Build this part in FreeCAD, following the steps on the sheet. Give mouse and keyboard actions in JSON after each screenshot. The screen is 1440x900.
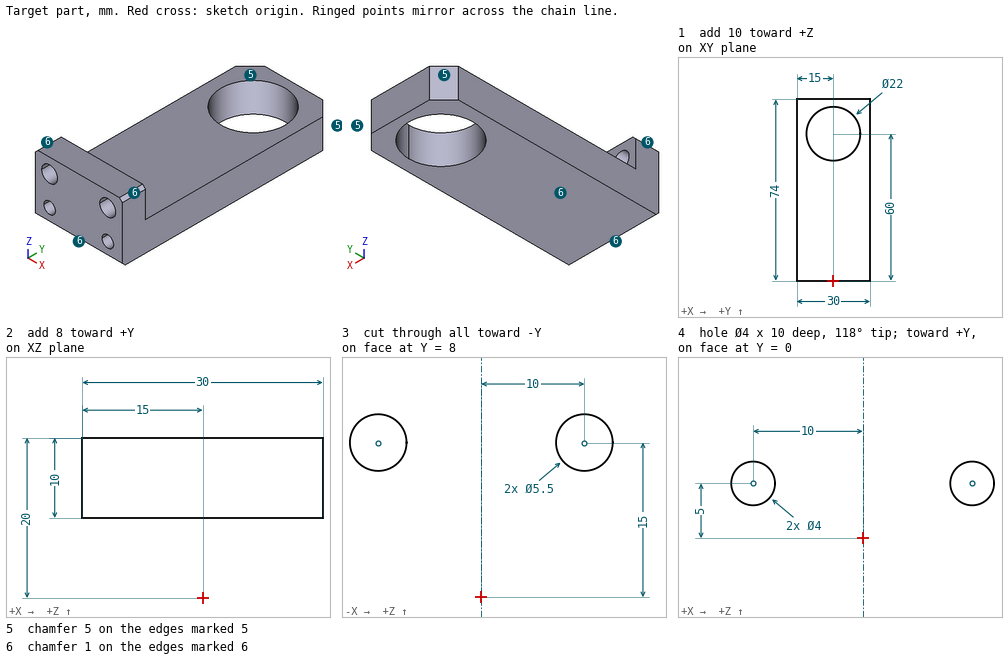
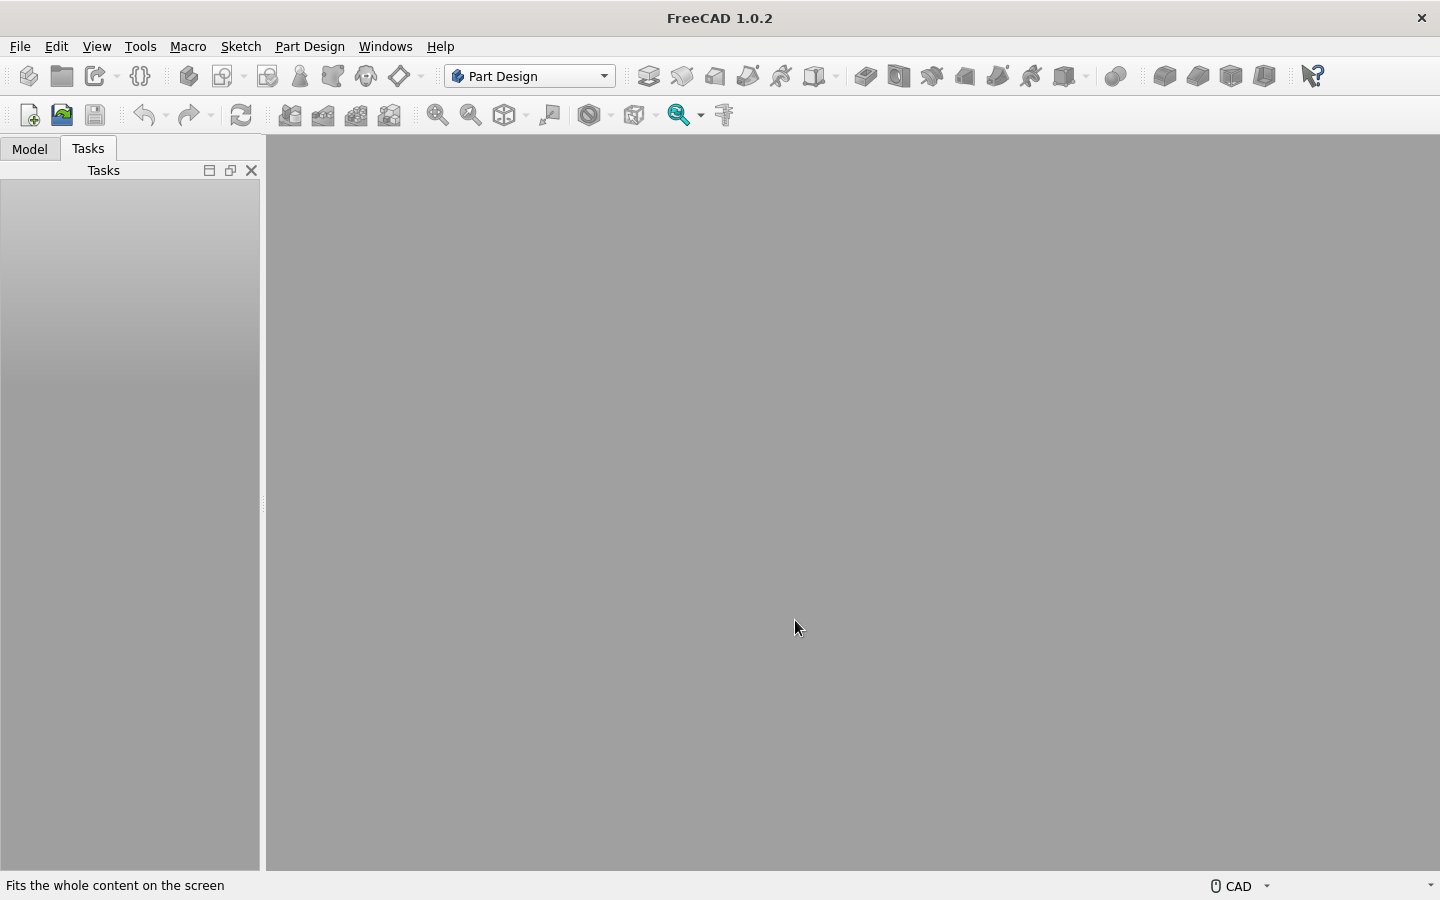
{"action": "left_click", "coordinate": [29, 116]}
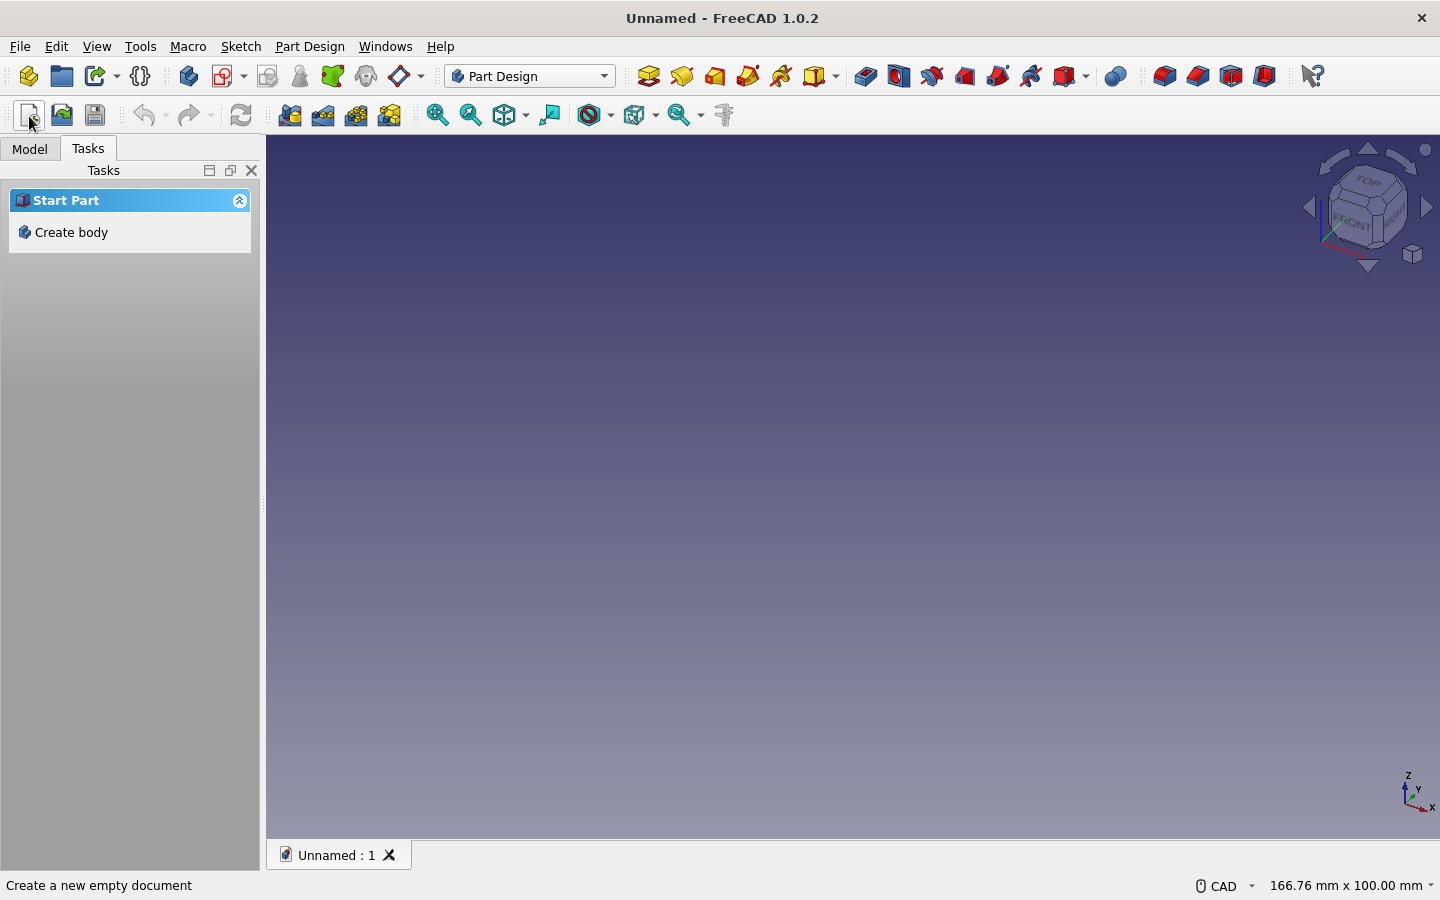
{"action": "left_click", "coordinate": [222, 76]}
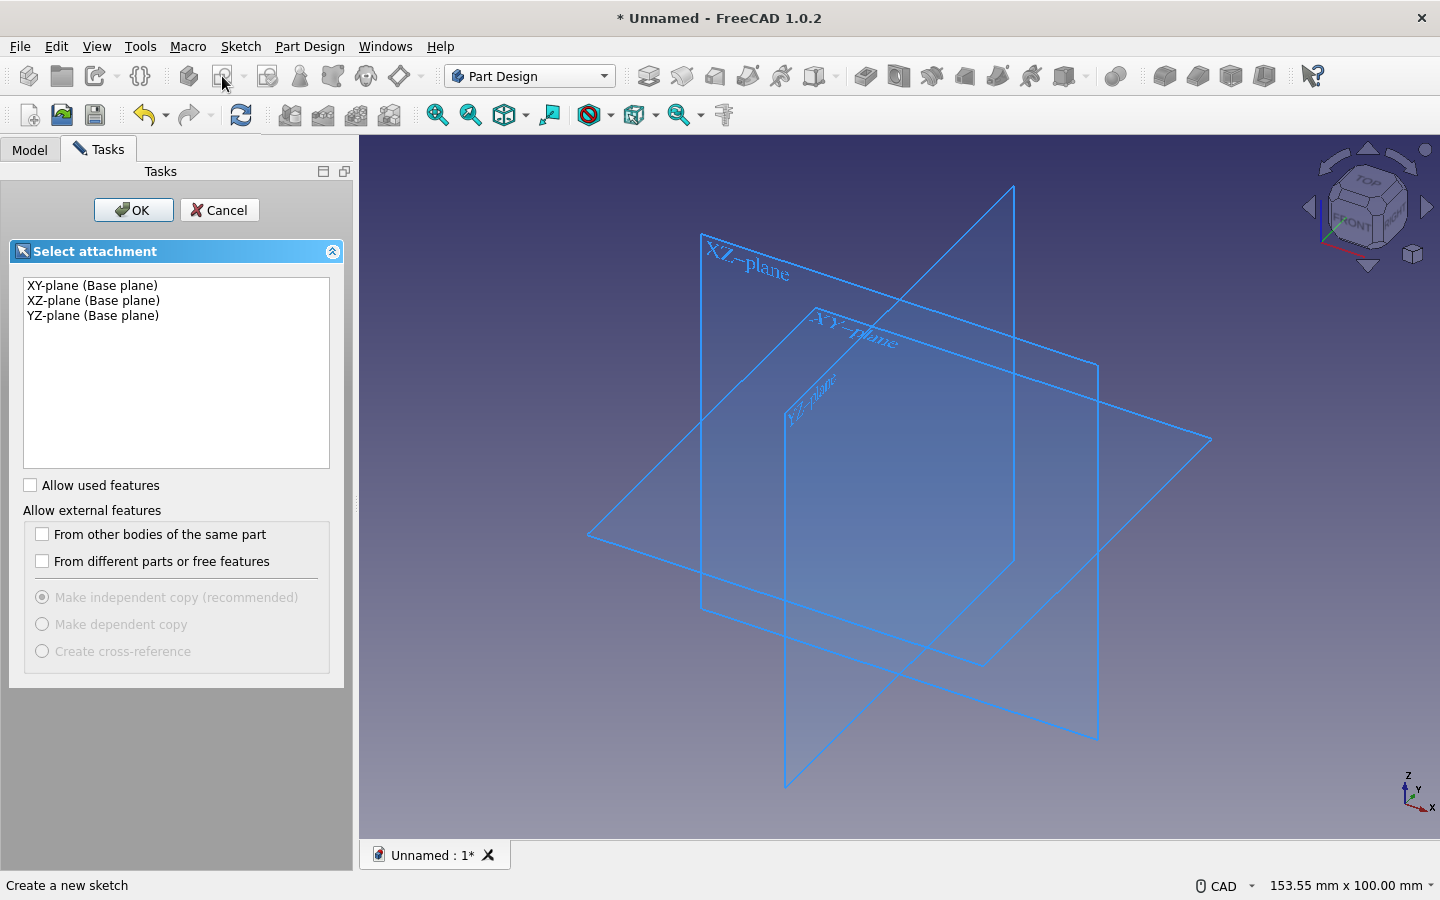
{"action": "left_click", "coordinate": [84, 286]}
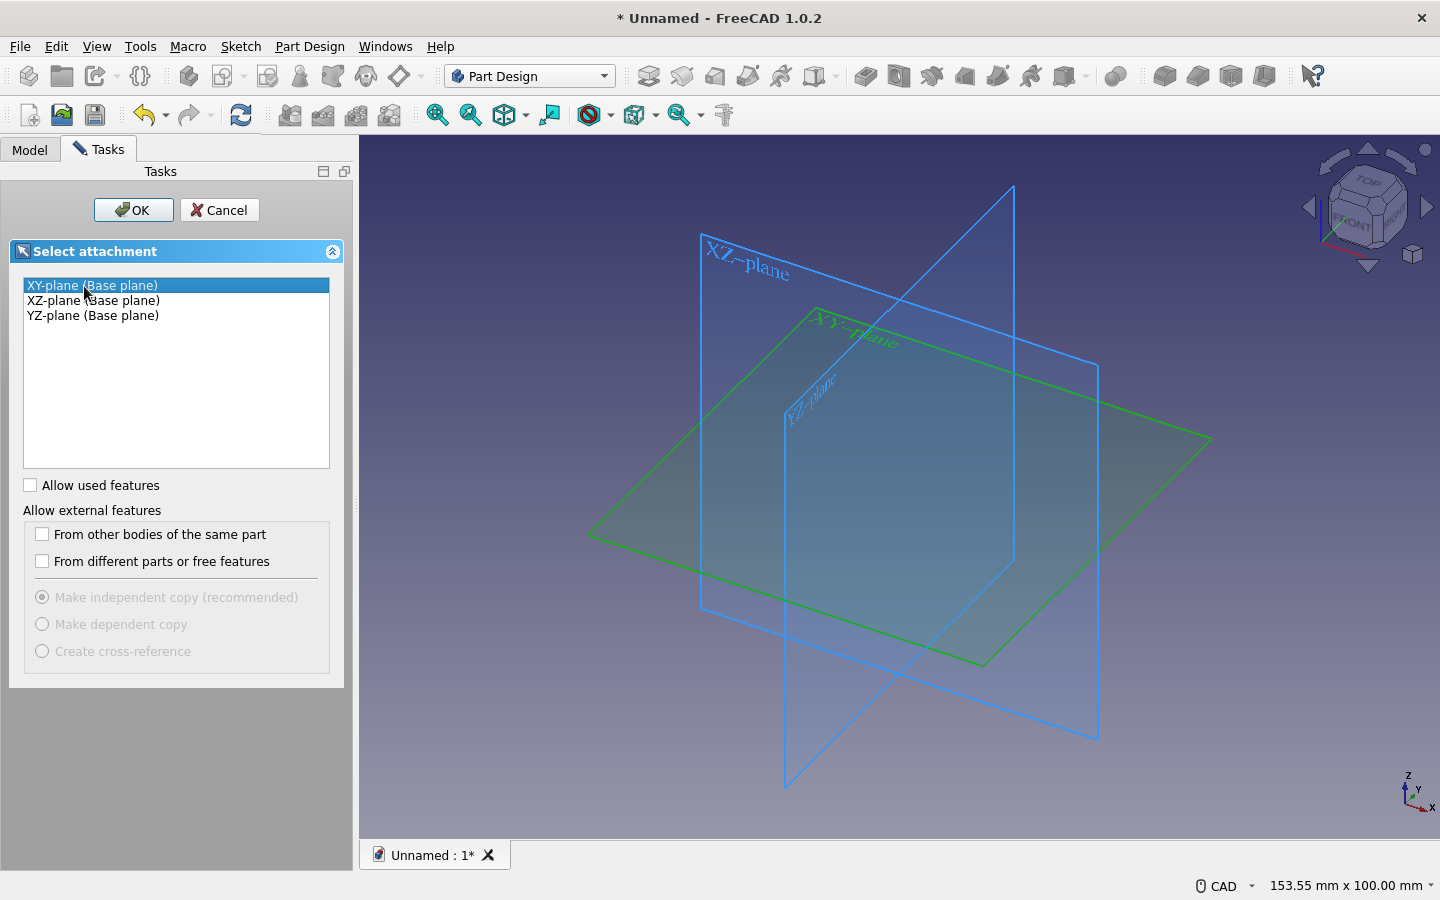
{"action": "left_click", "coordinate": [134, 210]}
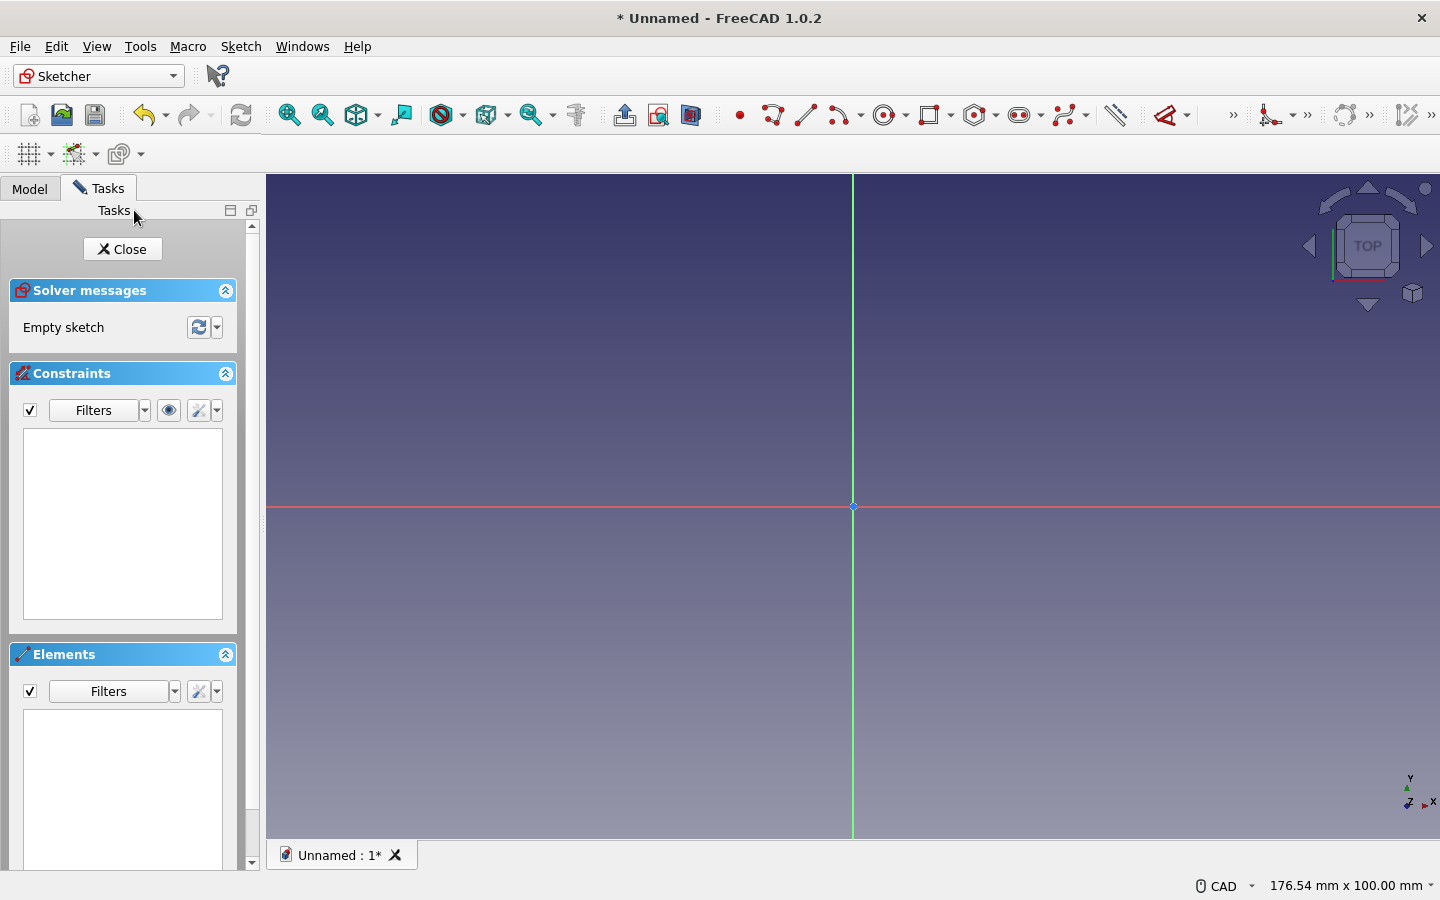
{"action": "scroll", "coordinate": [645, 811], "scroll_direction": "down", "scroll_amount": 2}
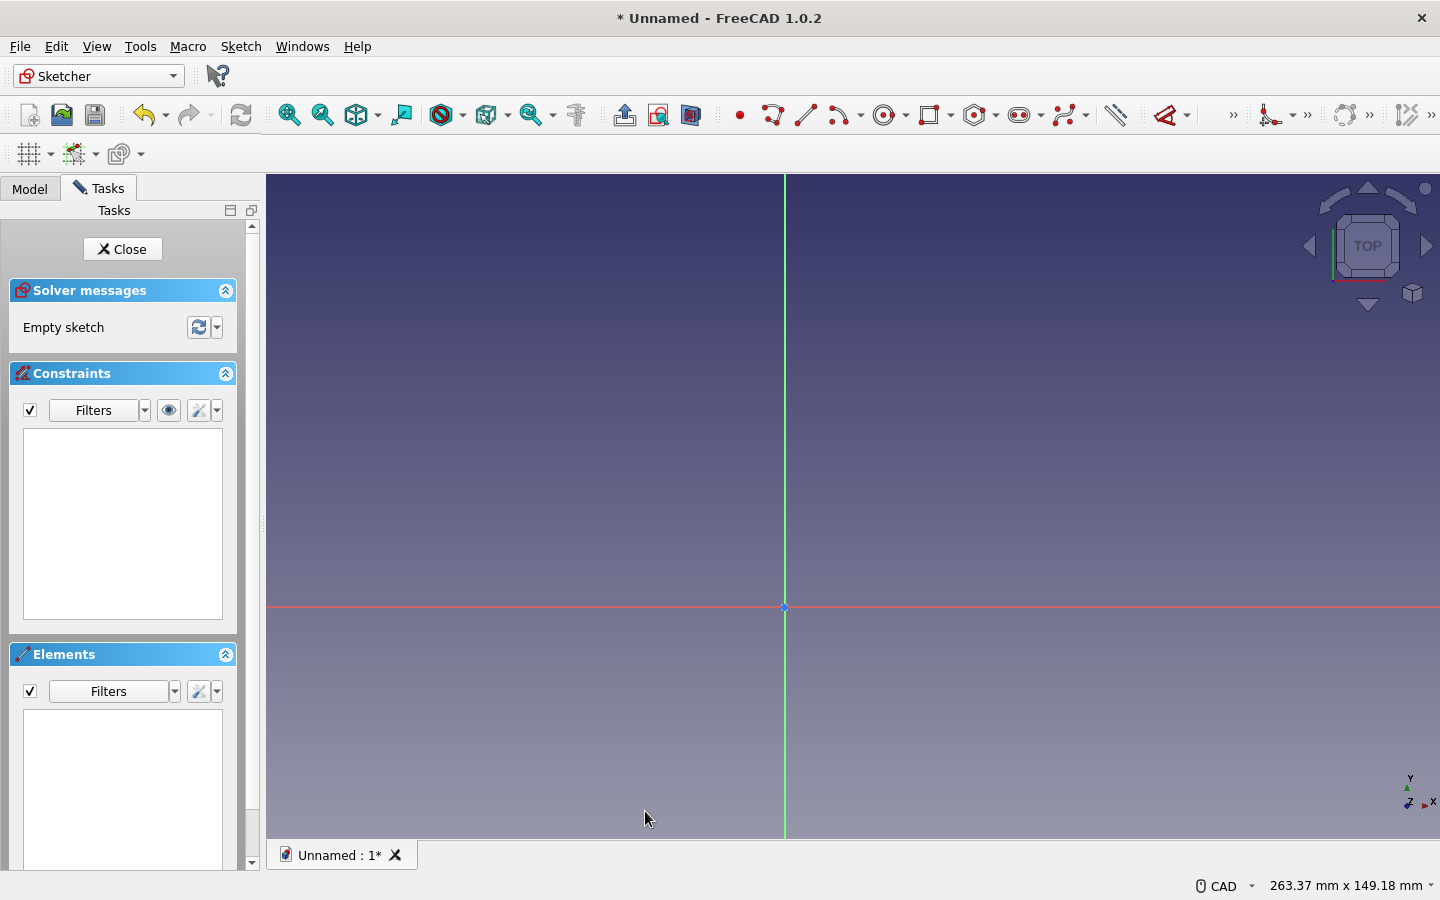
{"action": "left_click", "coordinate": [928, 116]}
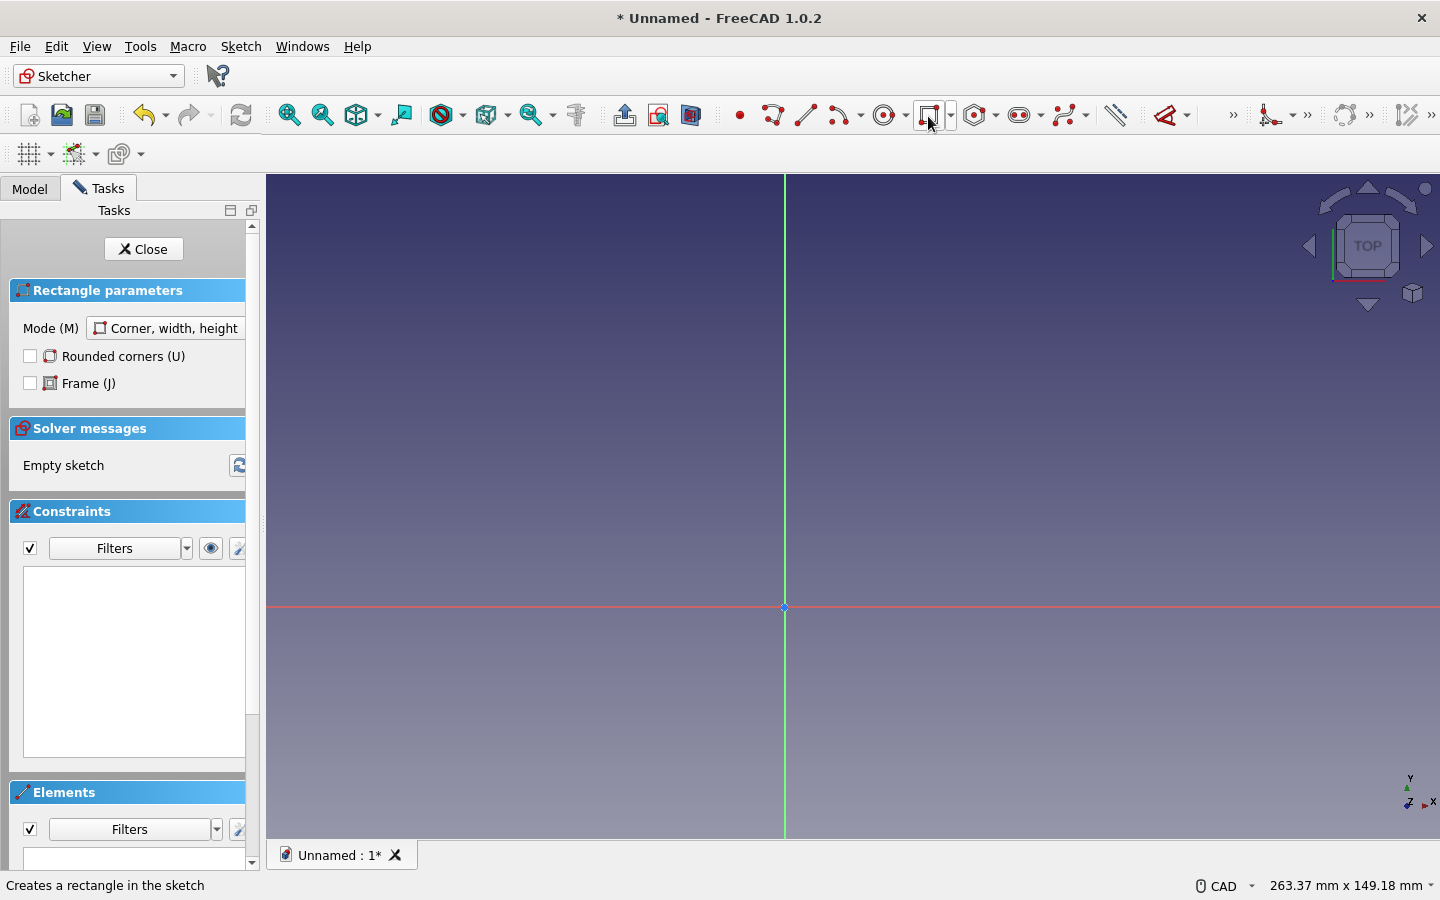
{"action": "left_click", "coordinate": [718, 277]}
{"action": "left_click", "coordinate": [851, 607]}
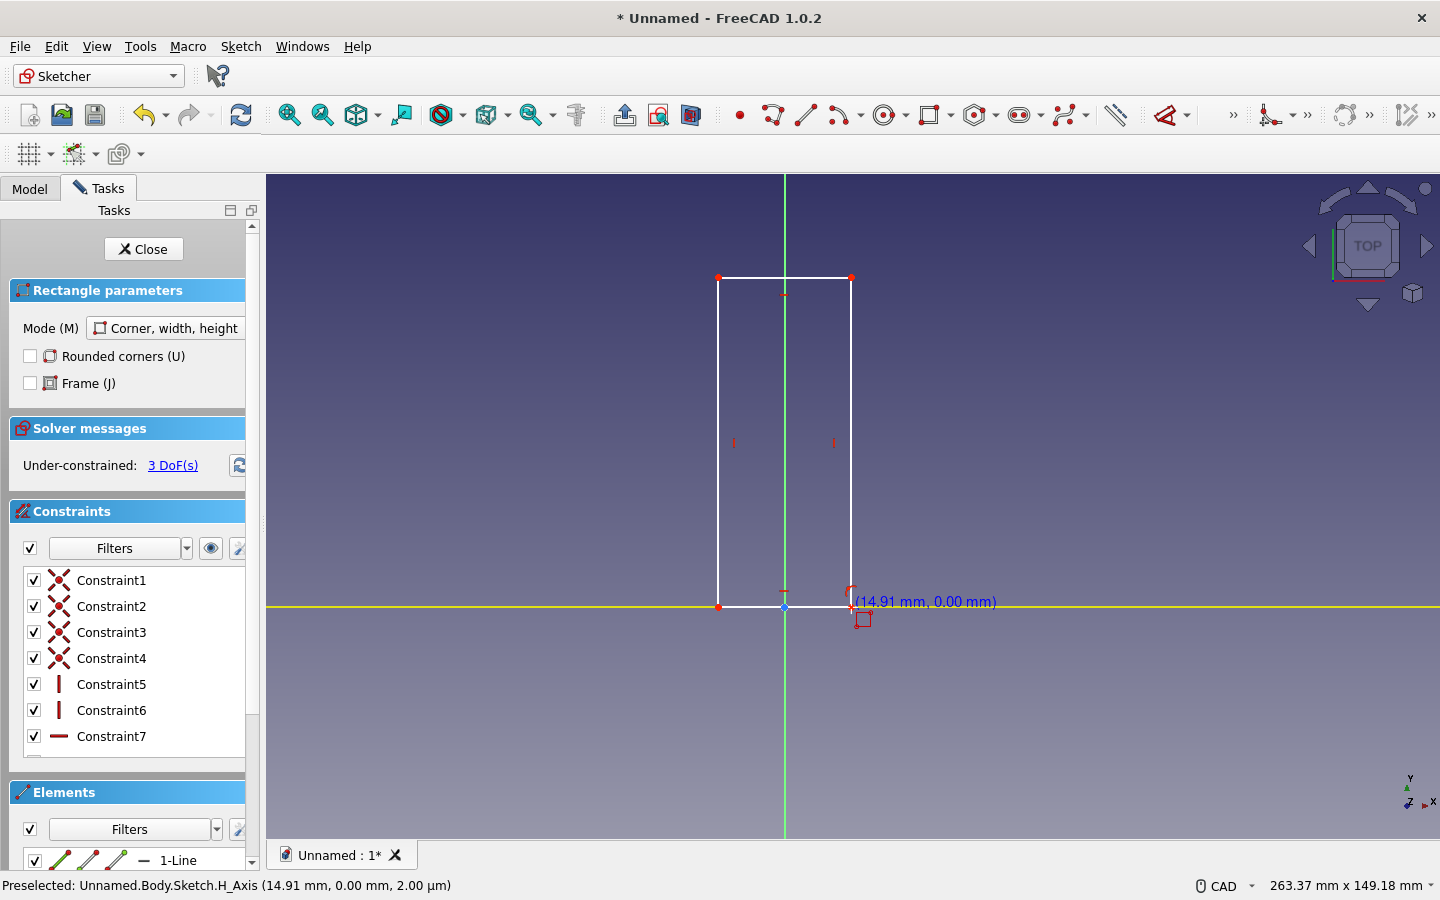
{"action": "left_click", "coordinate": [884, 116]}